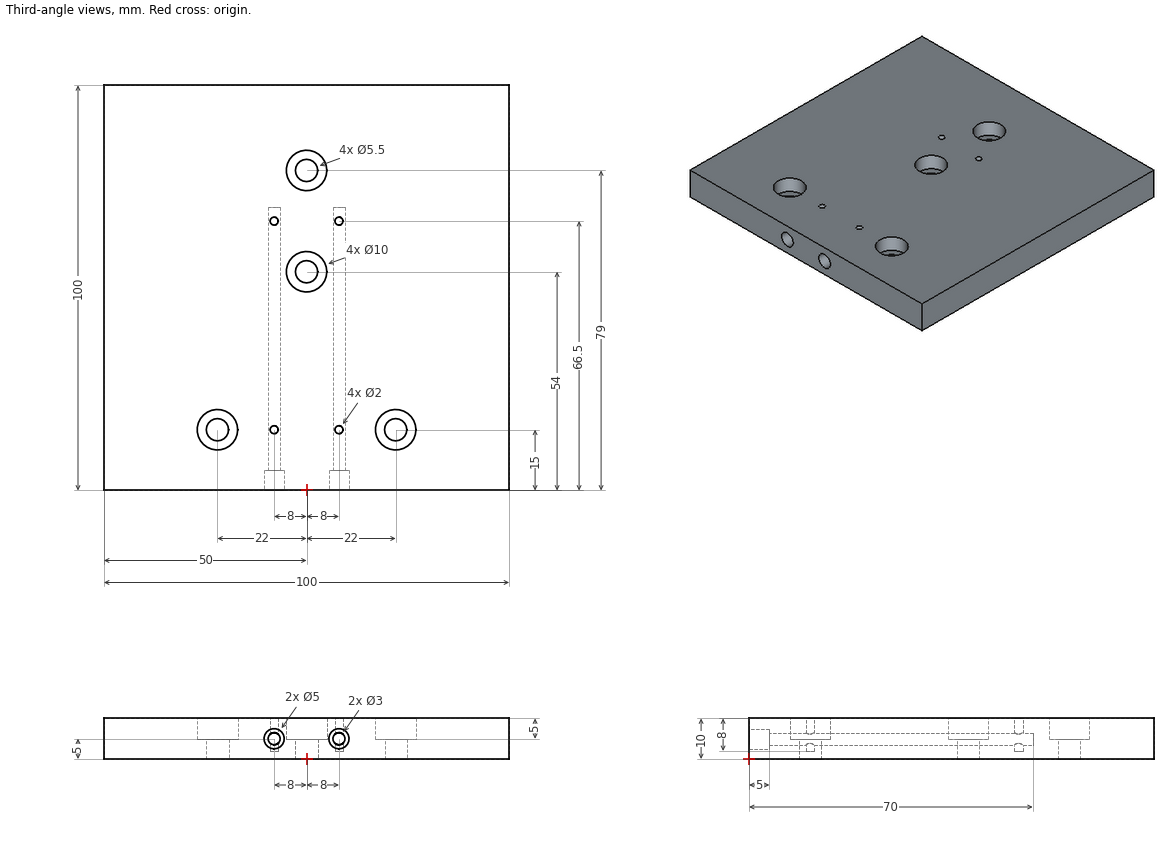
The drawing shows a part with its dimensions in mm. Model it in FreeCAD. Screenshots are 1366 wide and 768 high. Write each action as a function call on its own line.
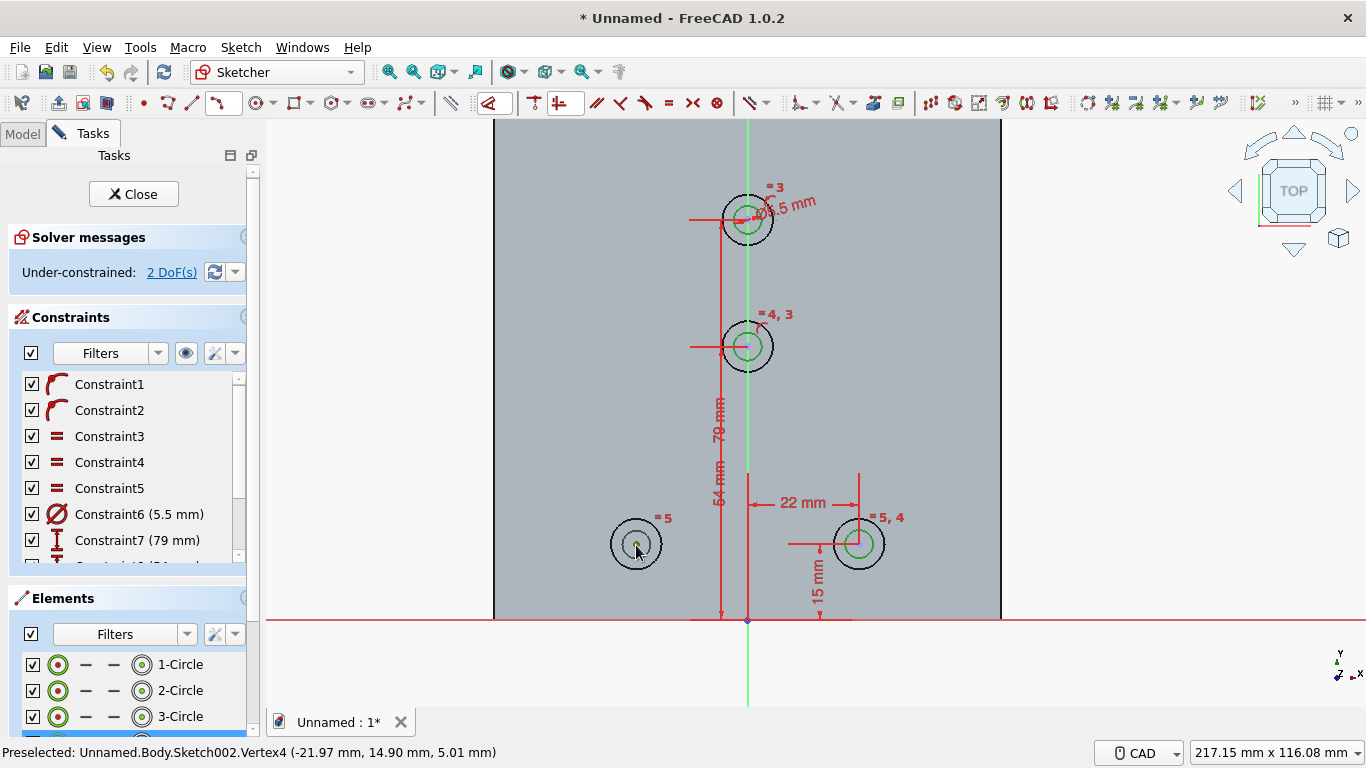
key(l)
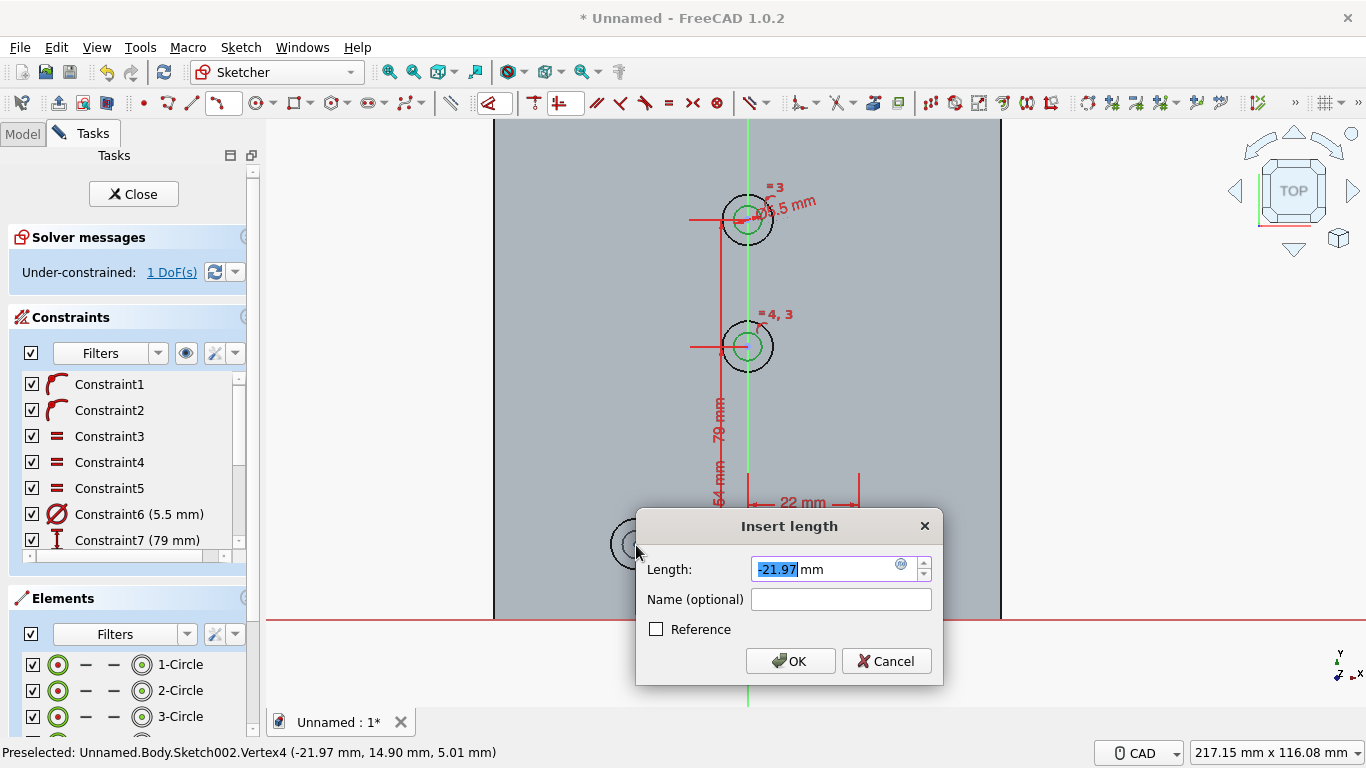
text(-22)
key(Return)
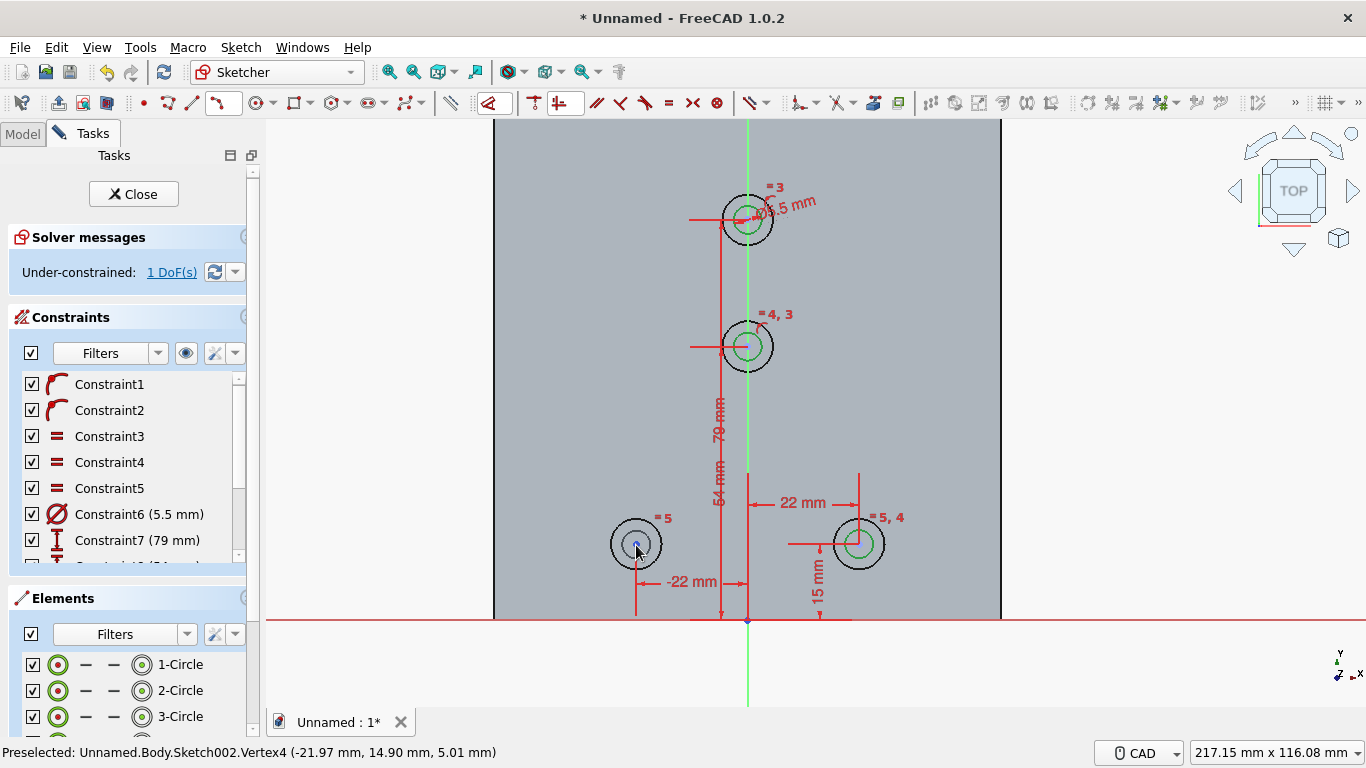
click(636, 545)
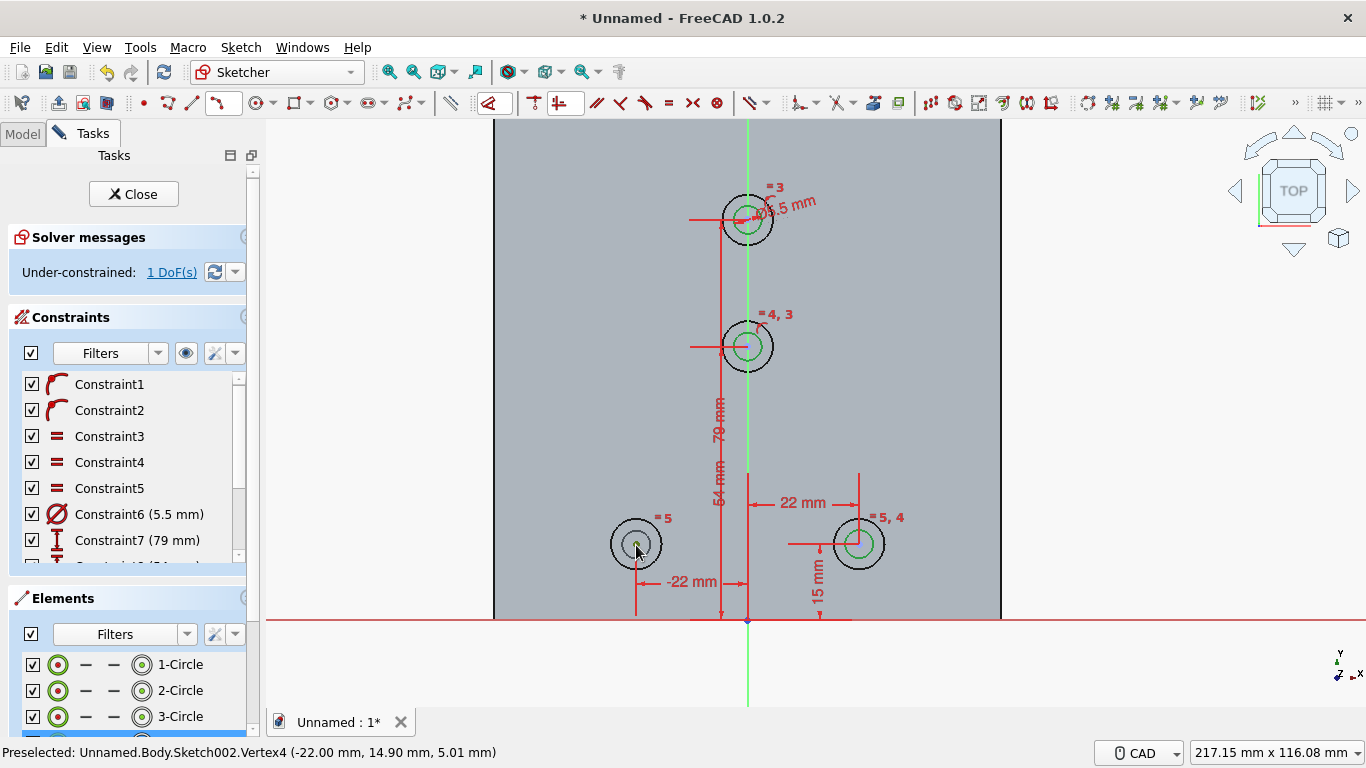
click(506, 104)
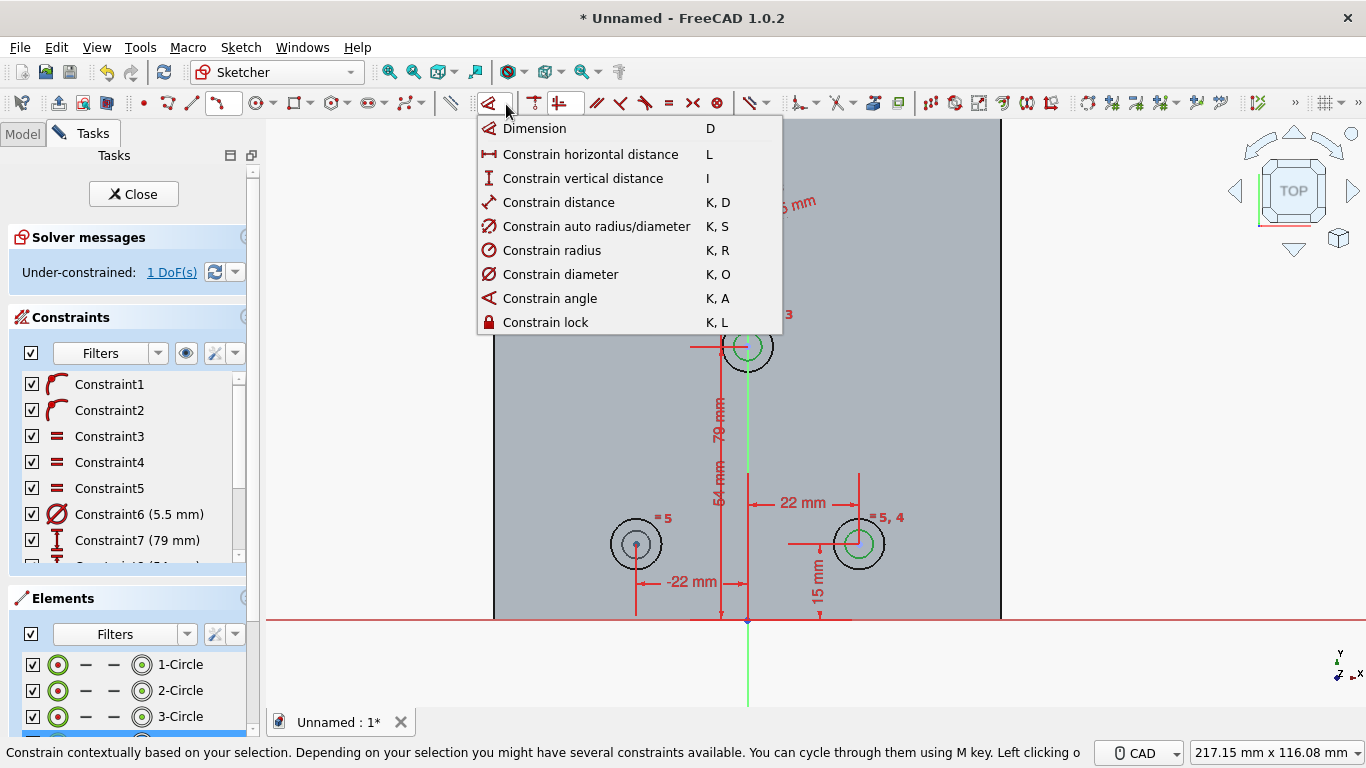
click(630, 178)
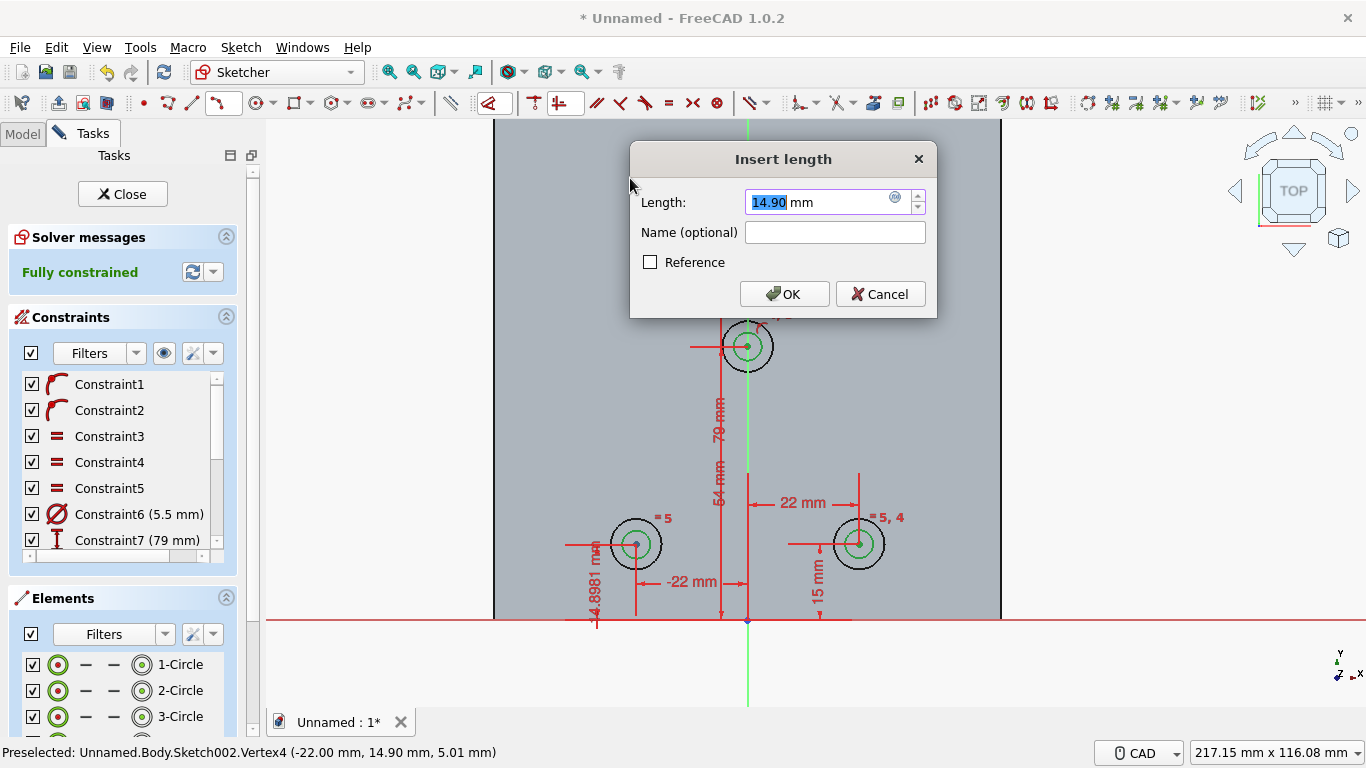
text(15)
key(Return)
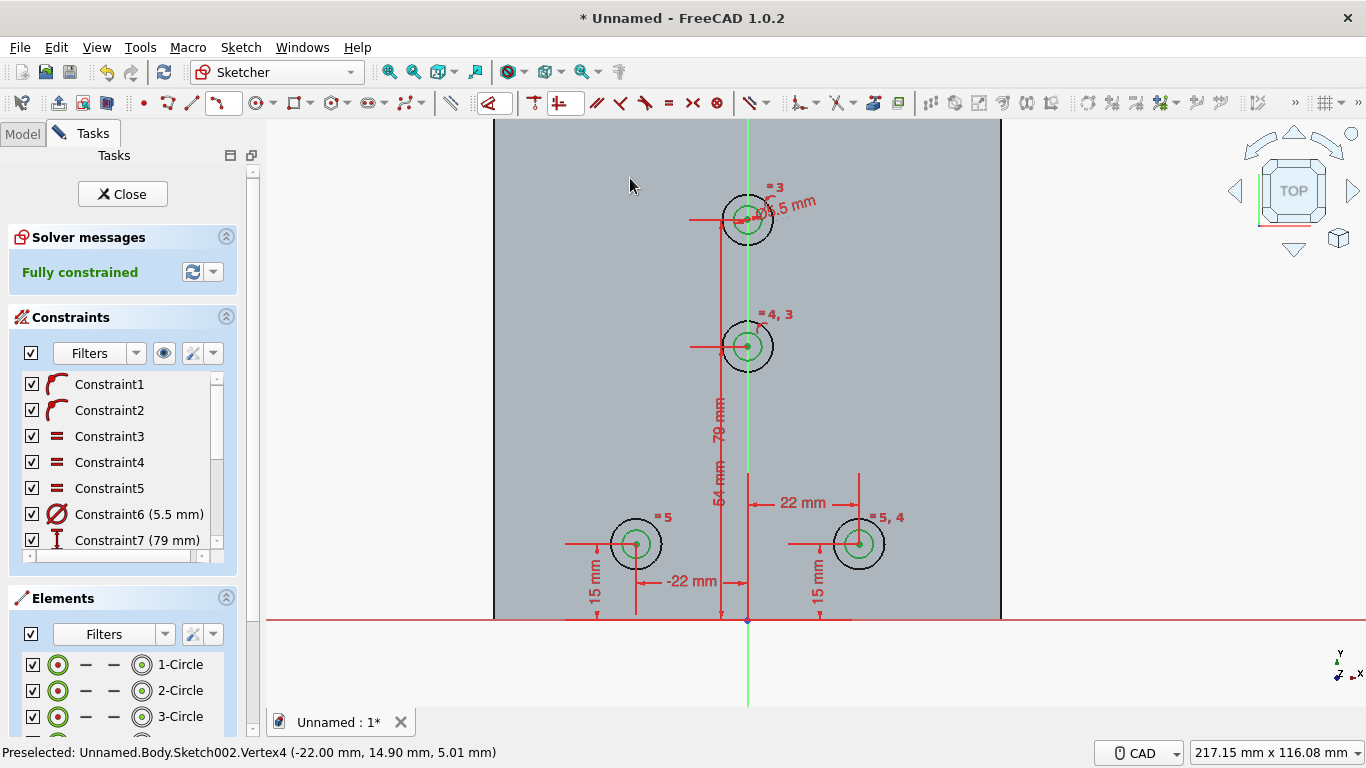
click(123, 194)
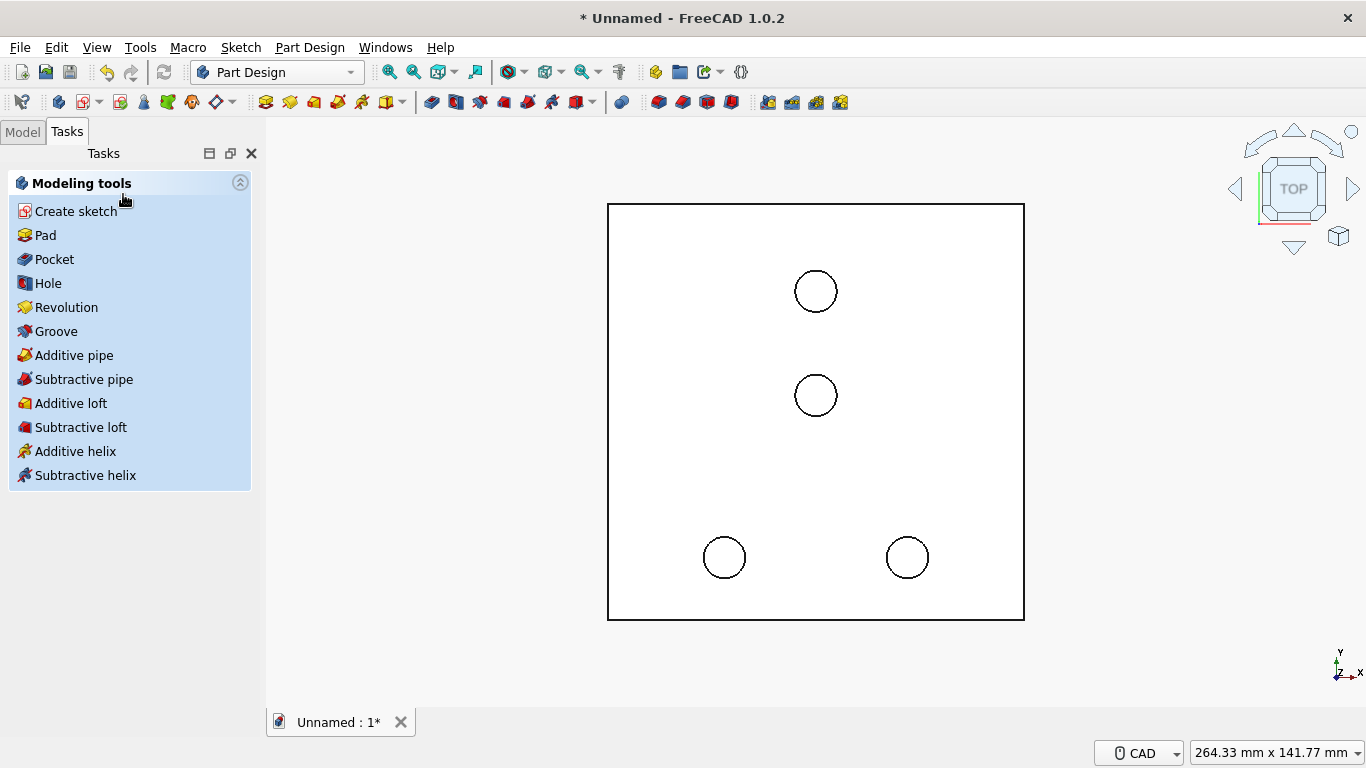
click(432, 102)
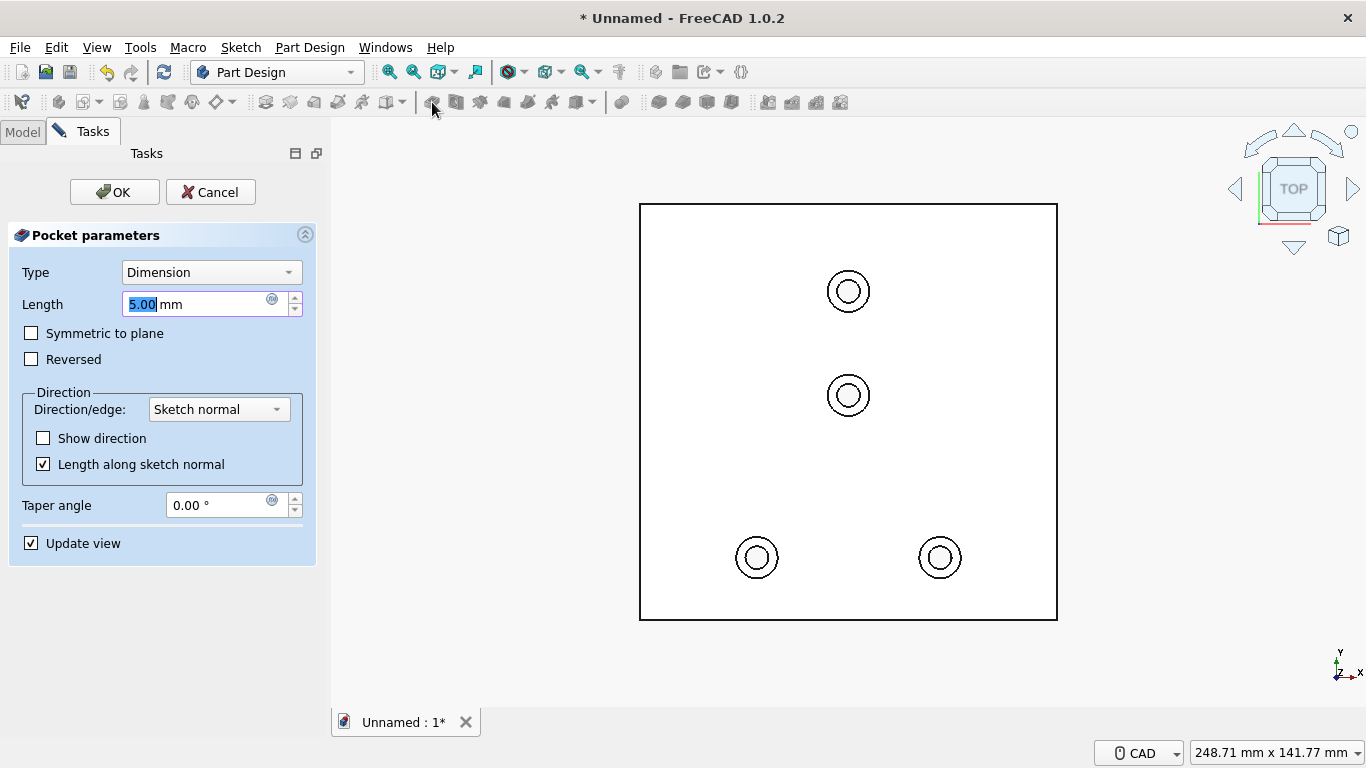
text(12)
key(Tab)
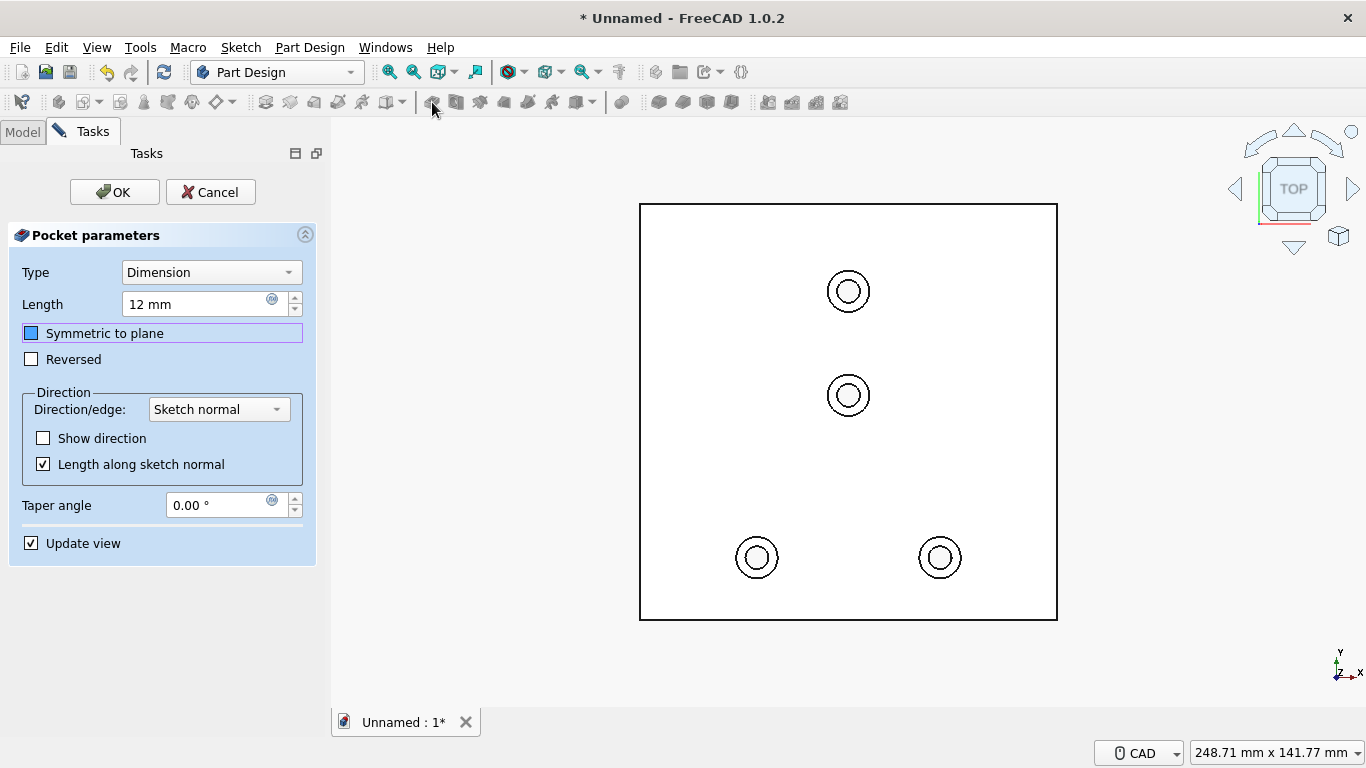
click(115, 192)